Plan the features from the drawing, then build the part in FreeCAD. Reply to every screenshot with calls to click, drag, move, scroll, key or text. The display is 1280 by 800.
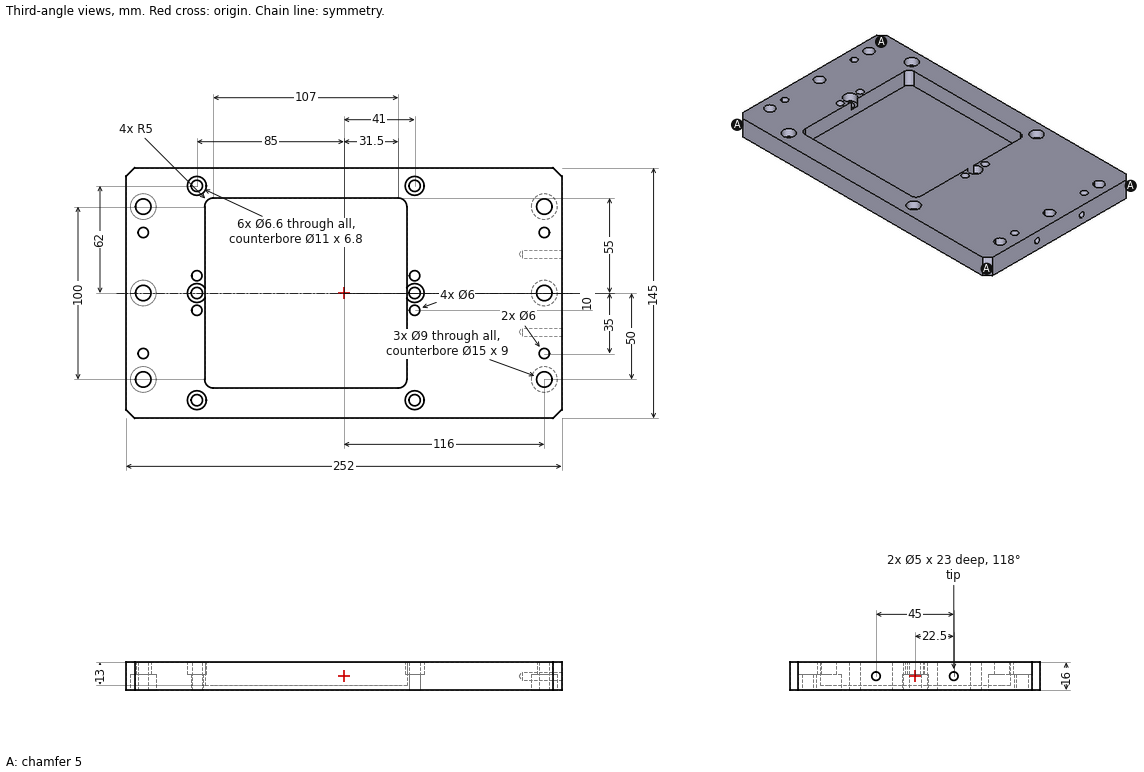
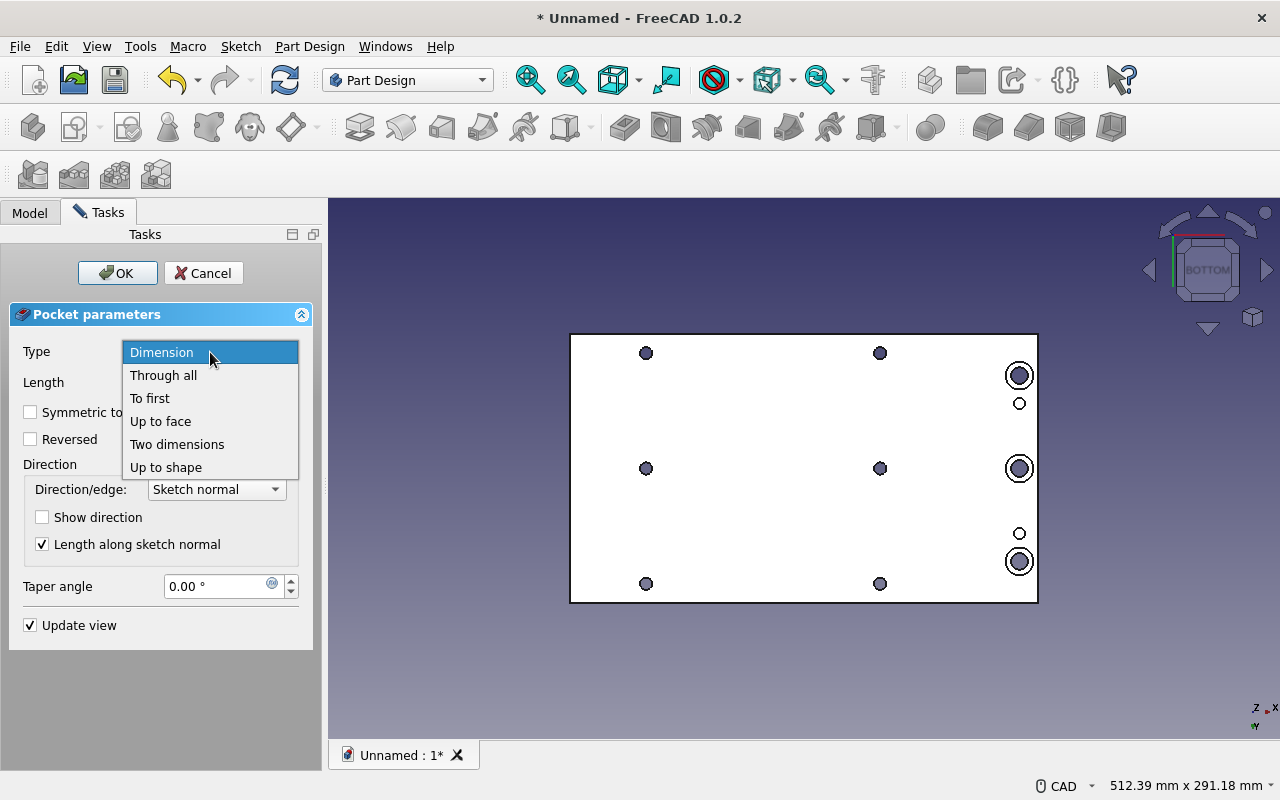
click(208, 376)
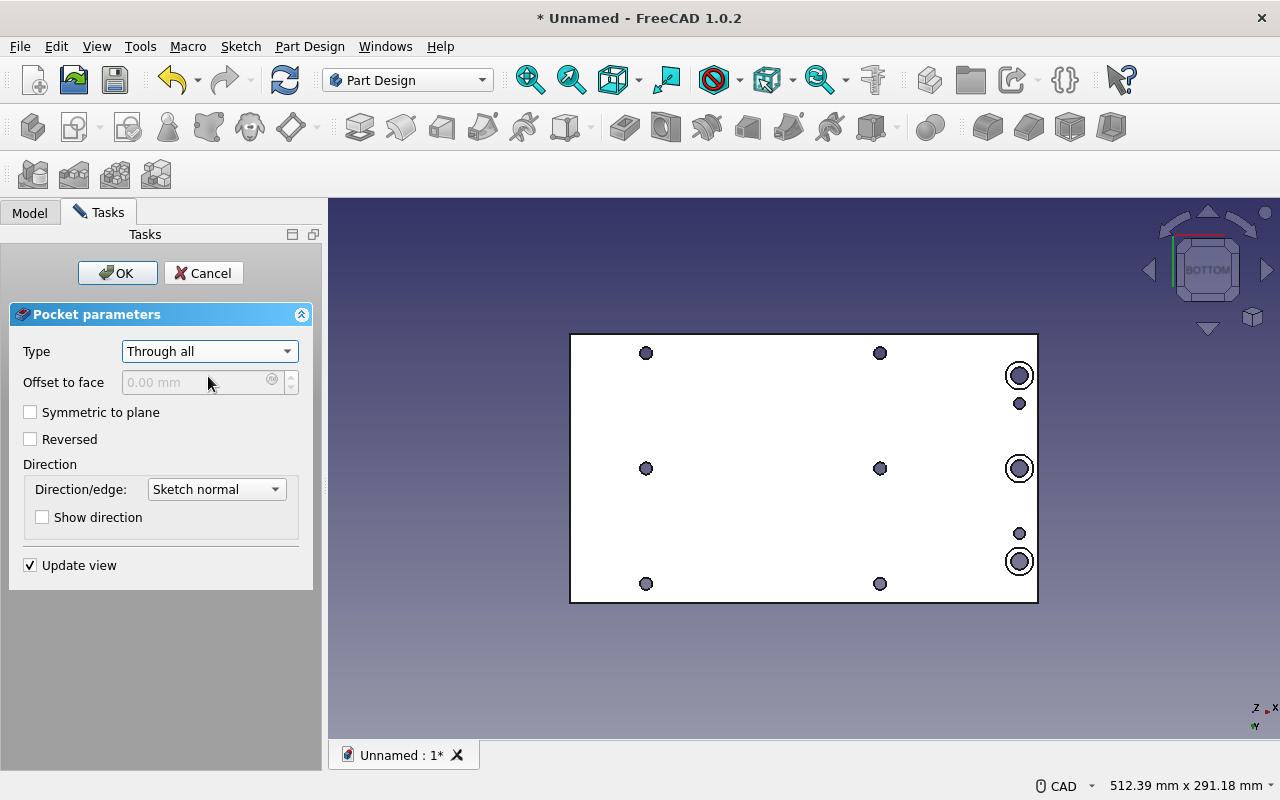
click(118, 273)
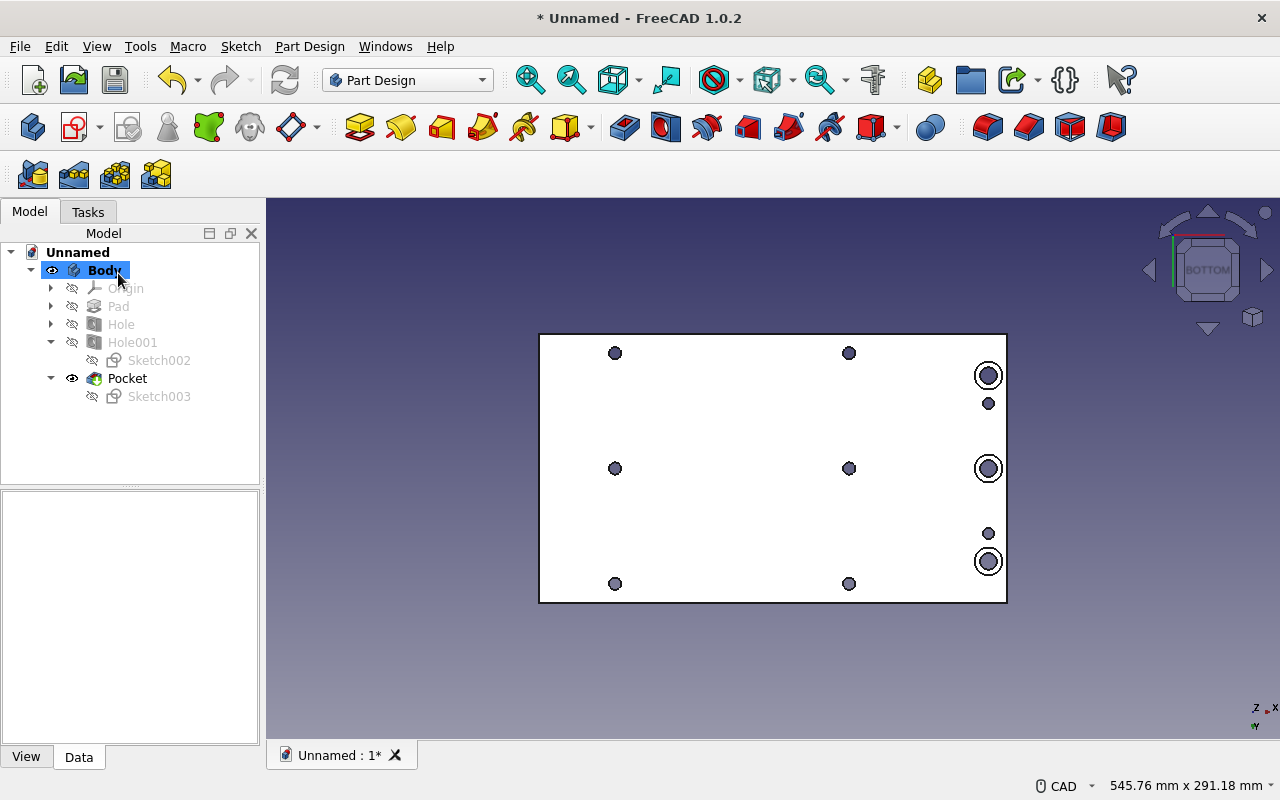
click(117, 342)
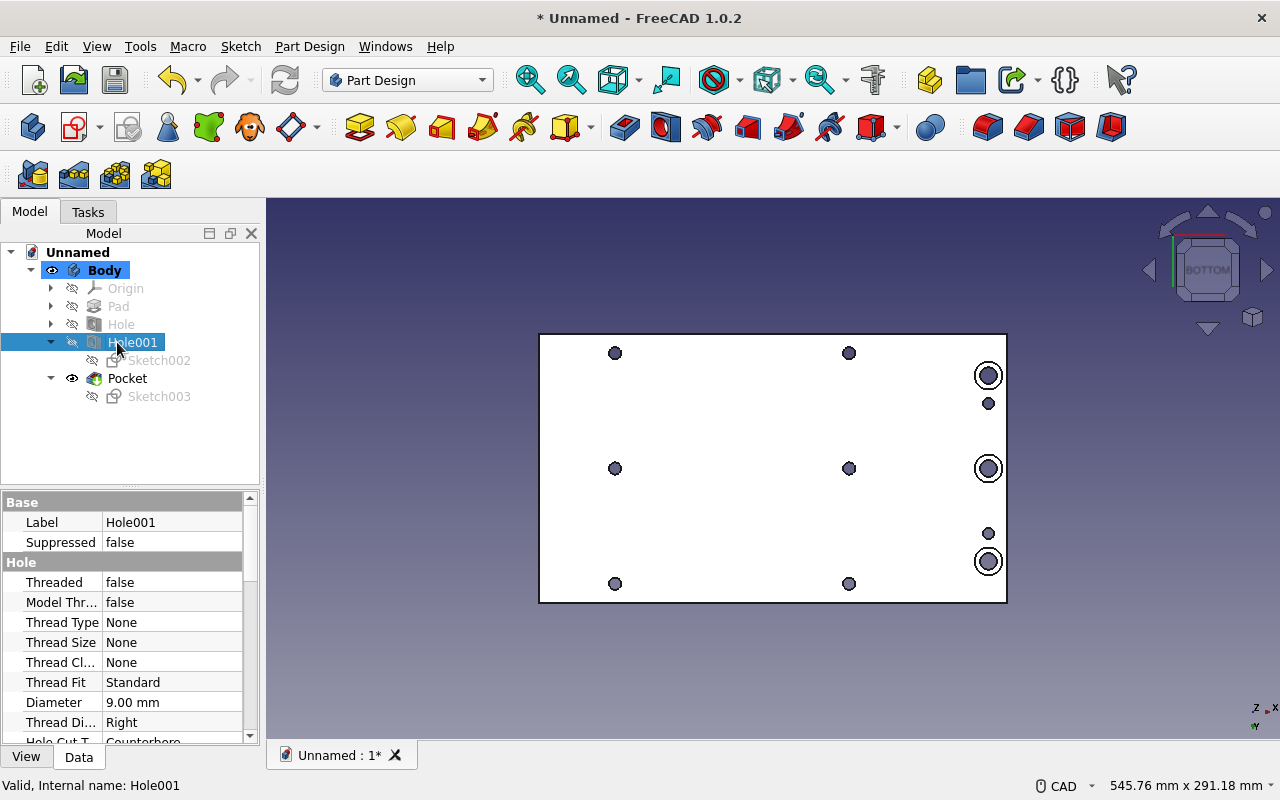
click(117, 378, ctrl)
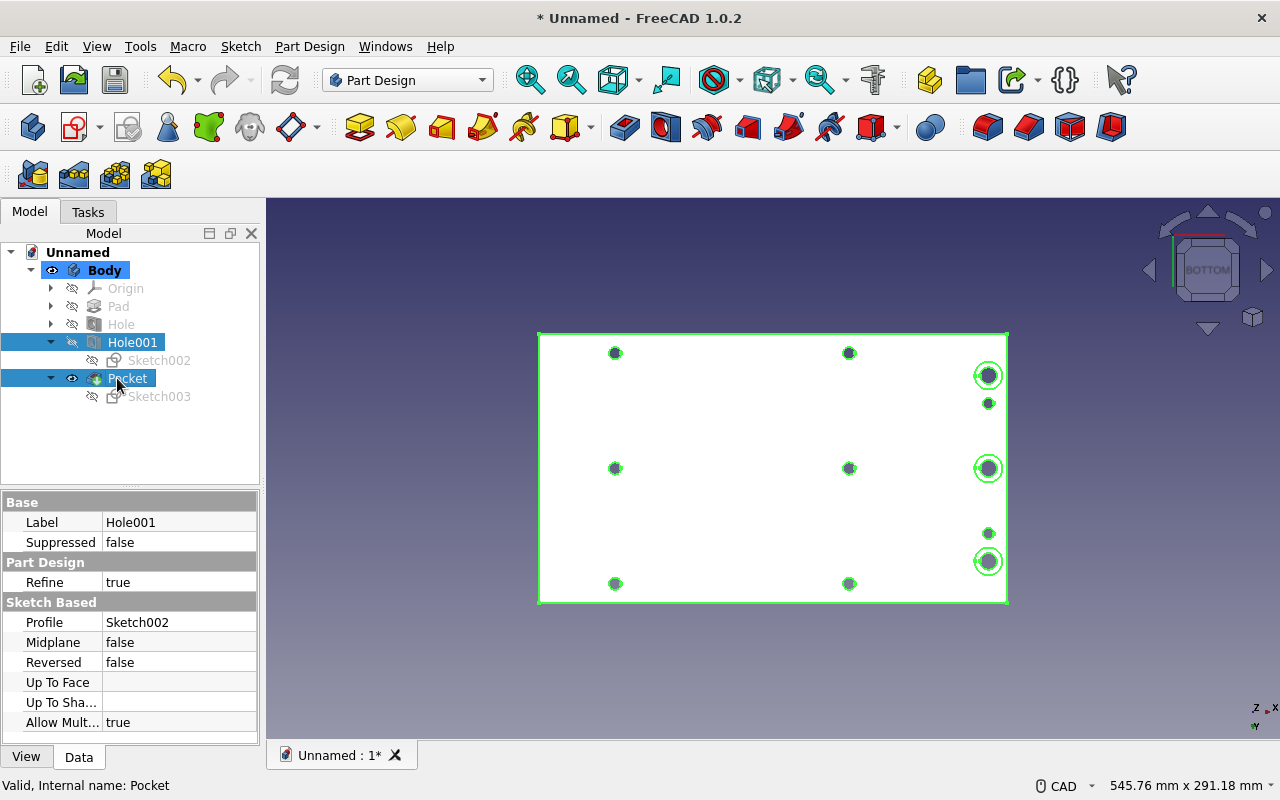
click(33, 174)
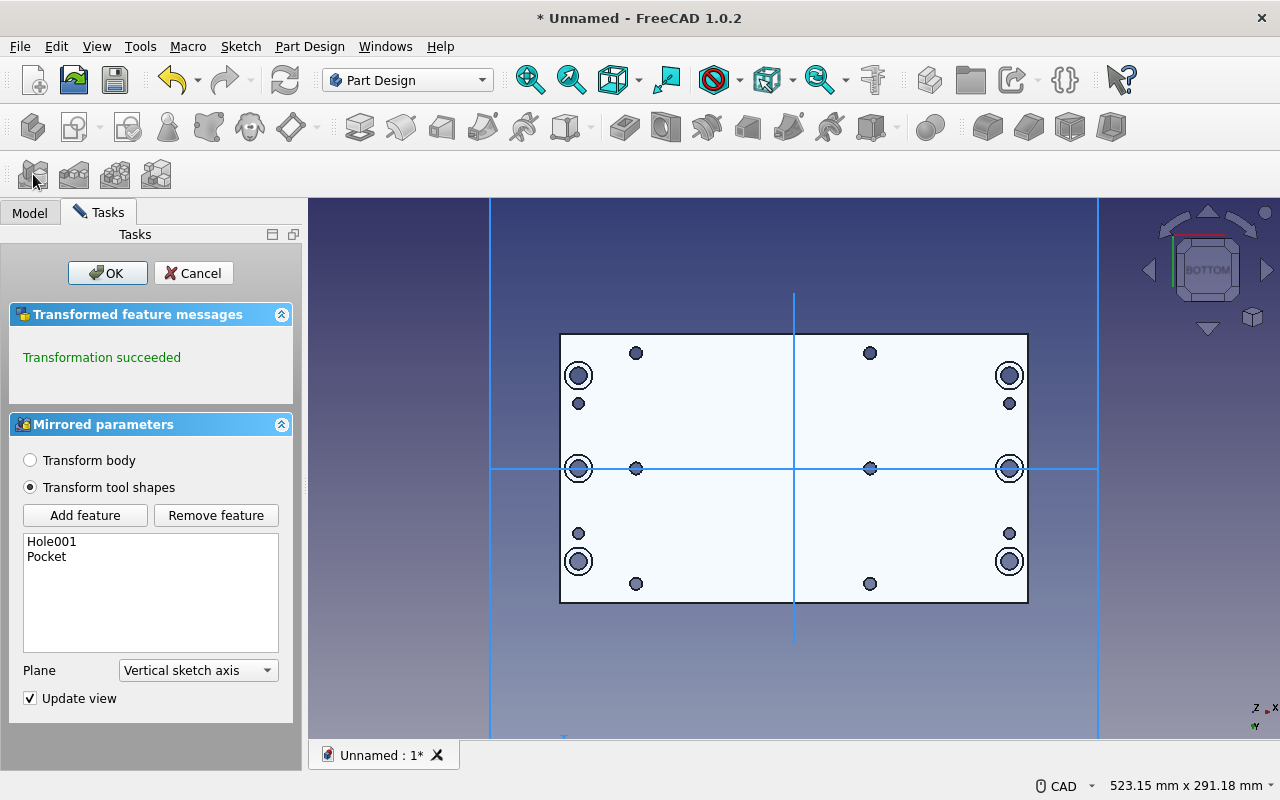
click(199, 670)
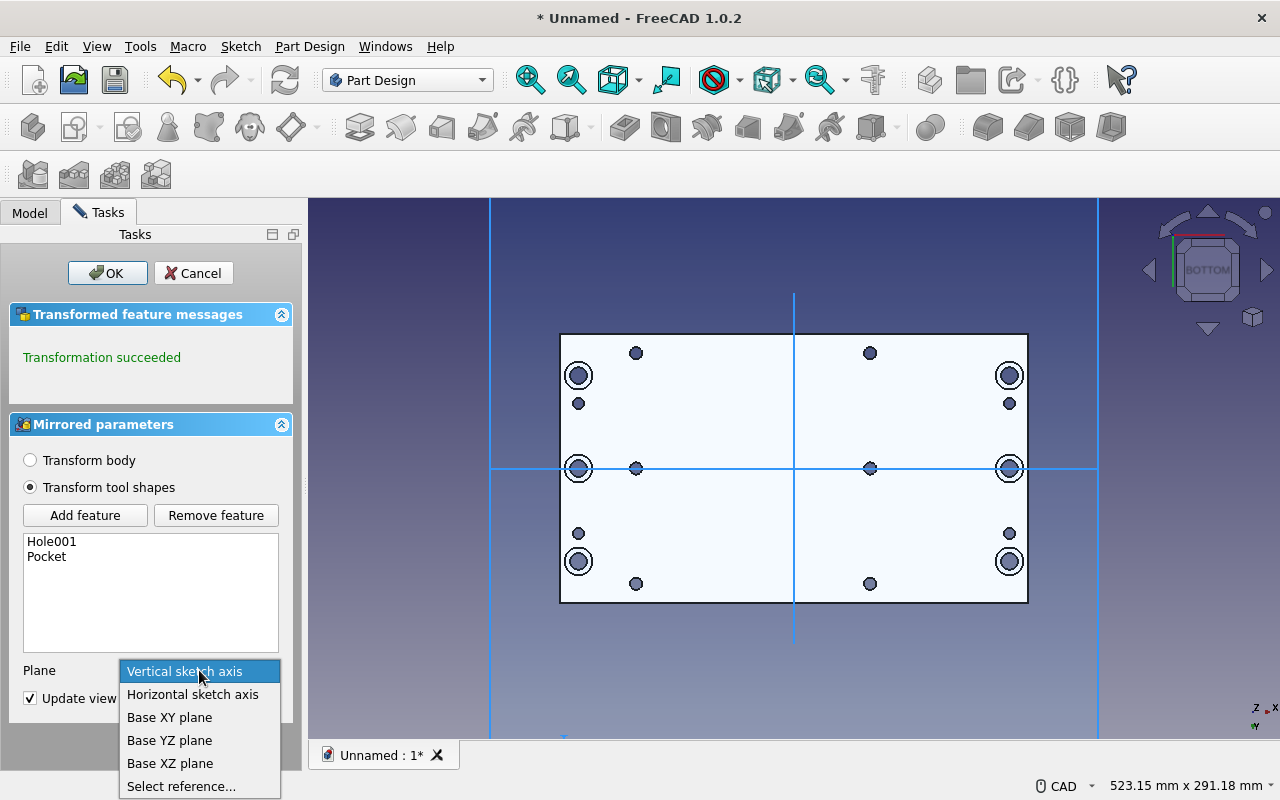
click(198, 740)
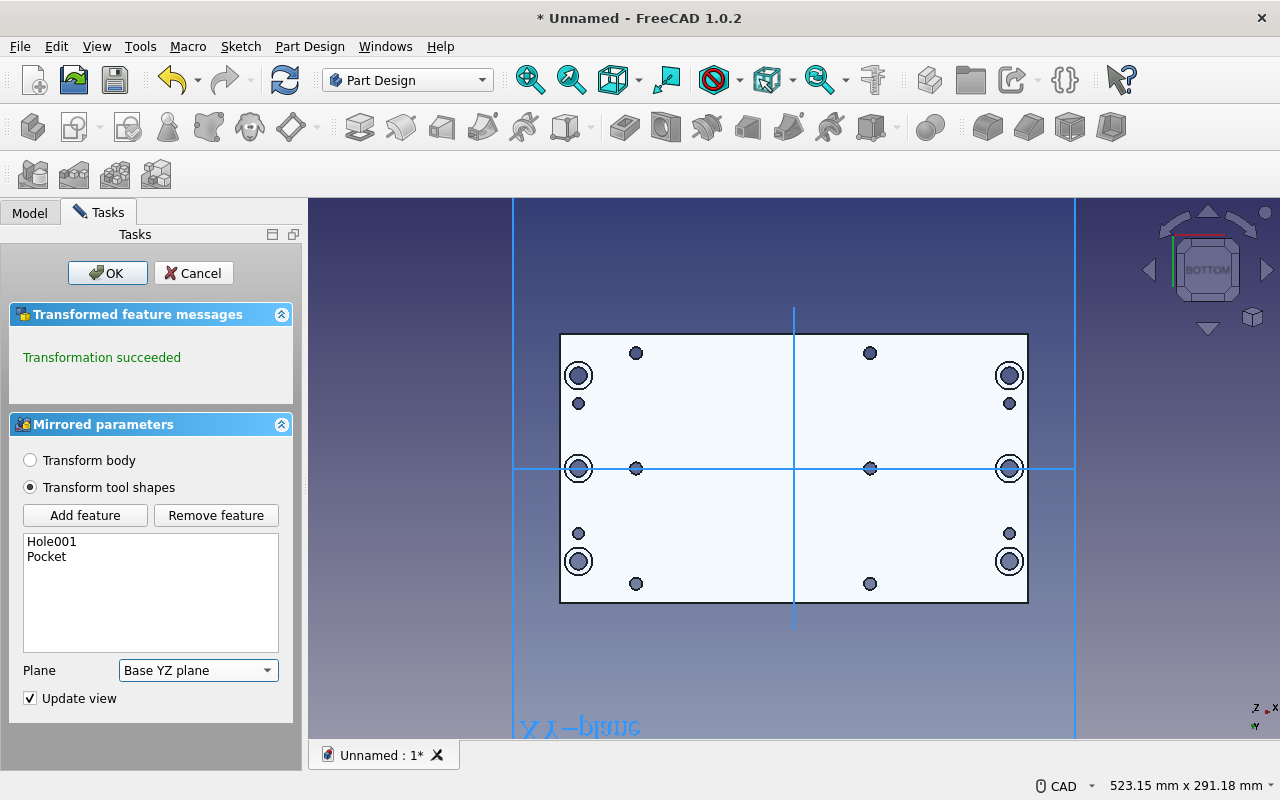
click(108, 273)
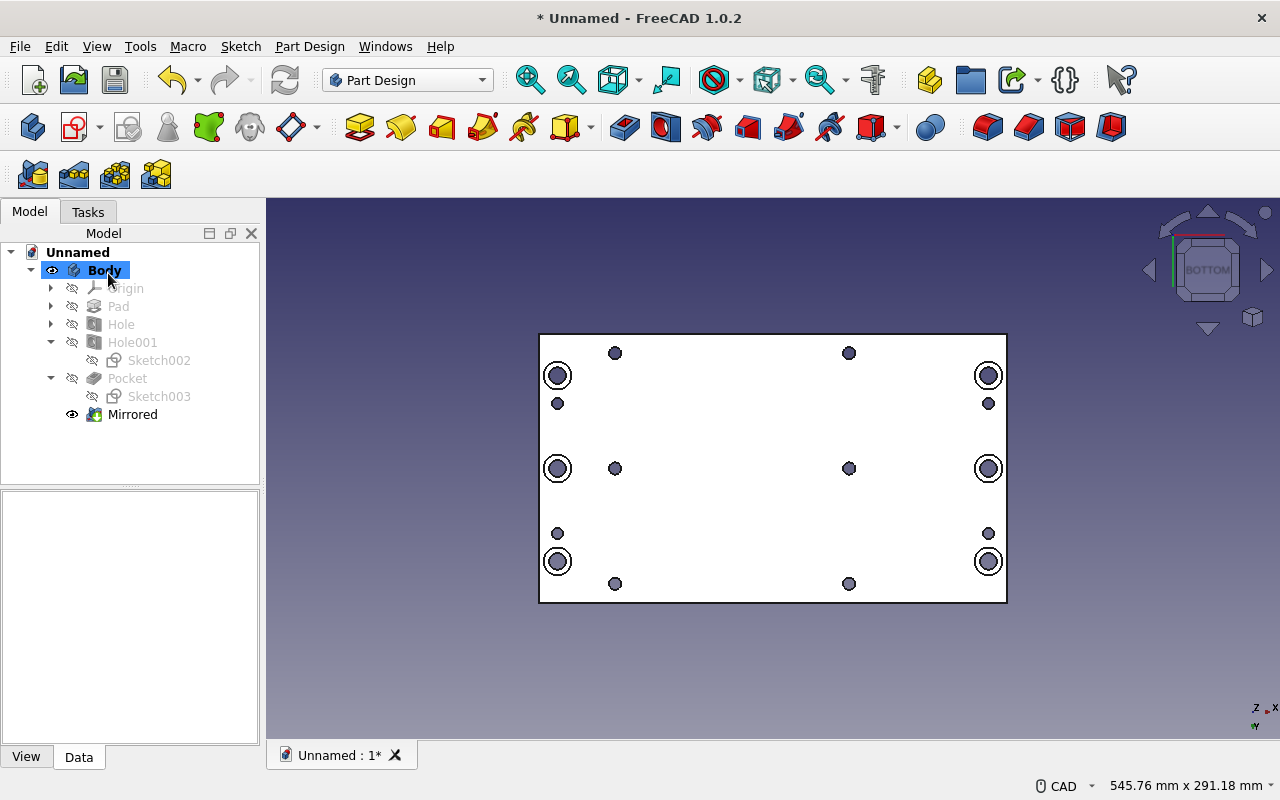
key(0)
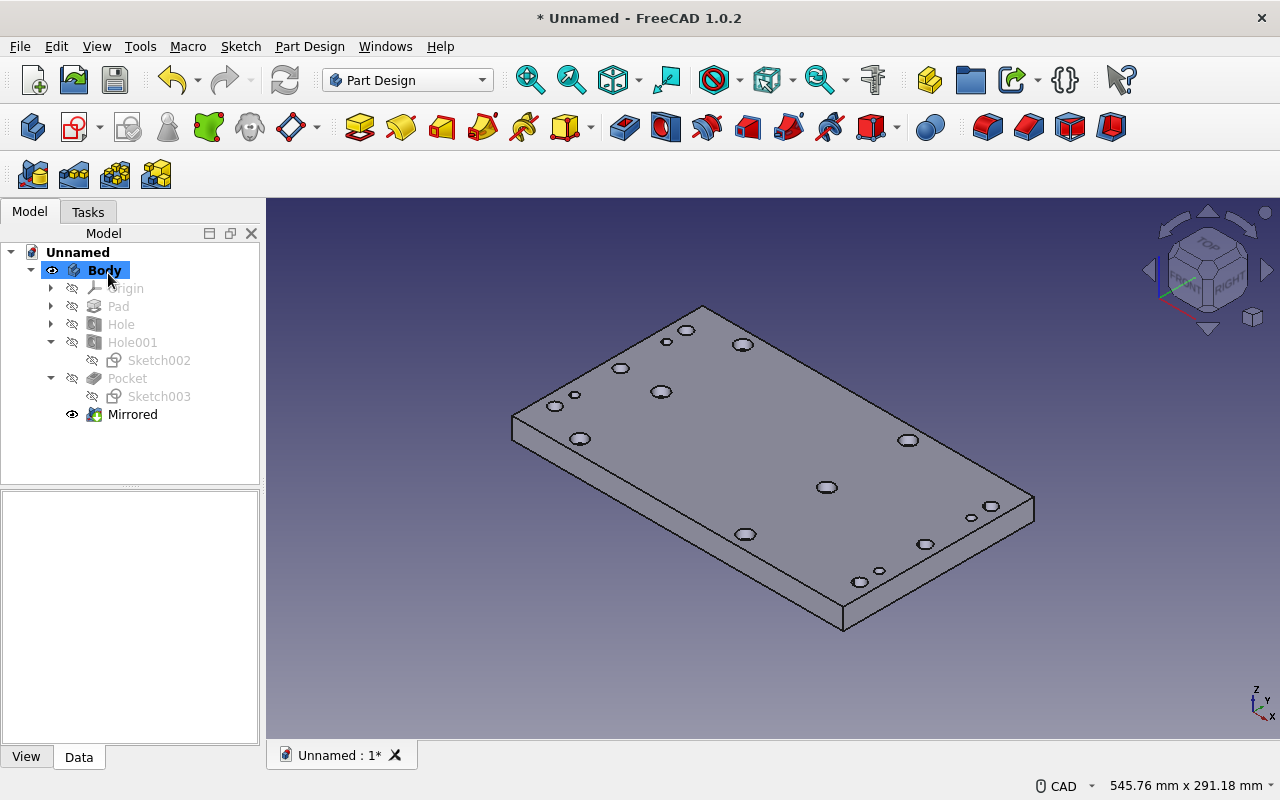
click(753, 412)